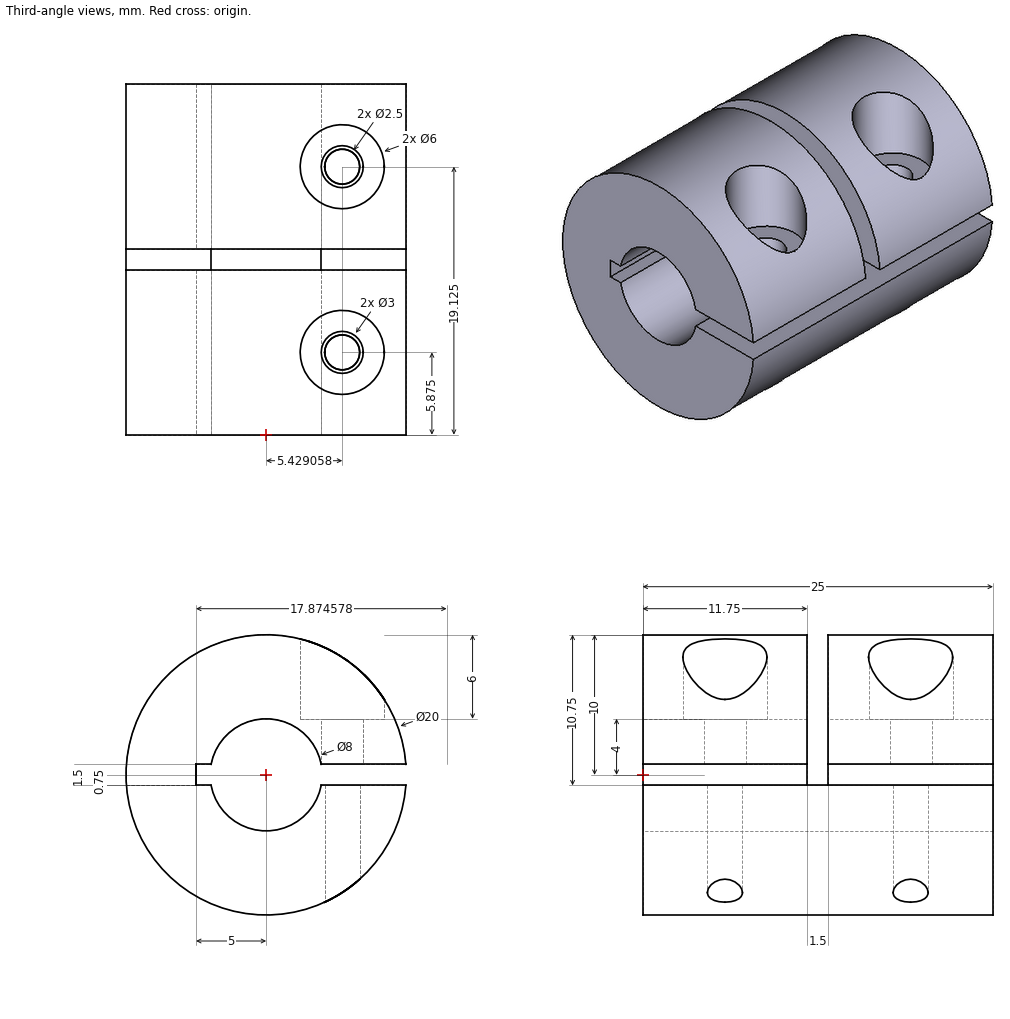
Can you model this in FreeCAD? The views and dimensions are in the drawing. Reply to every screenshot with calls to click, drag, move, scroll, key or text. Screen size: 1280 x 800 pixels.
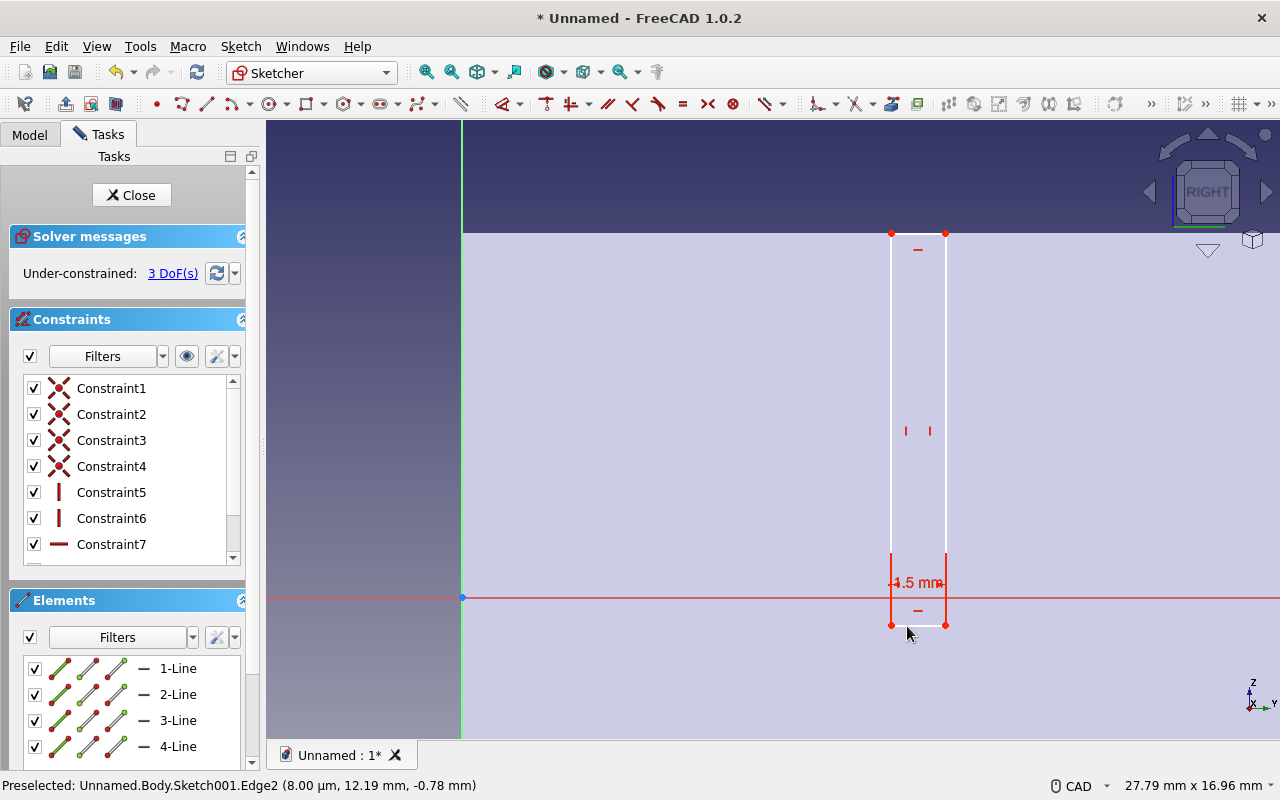
click(891, 234)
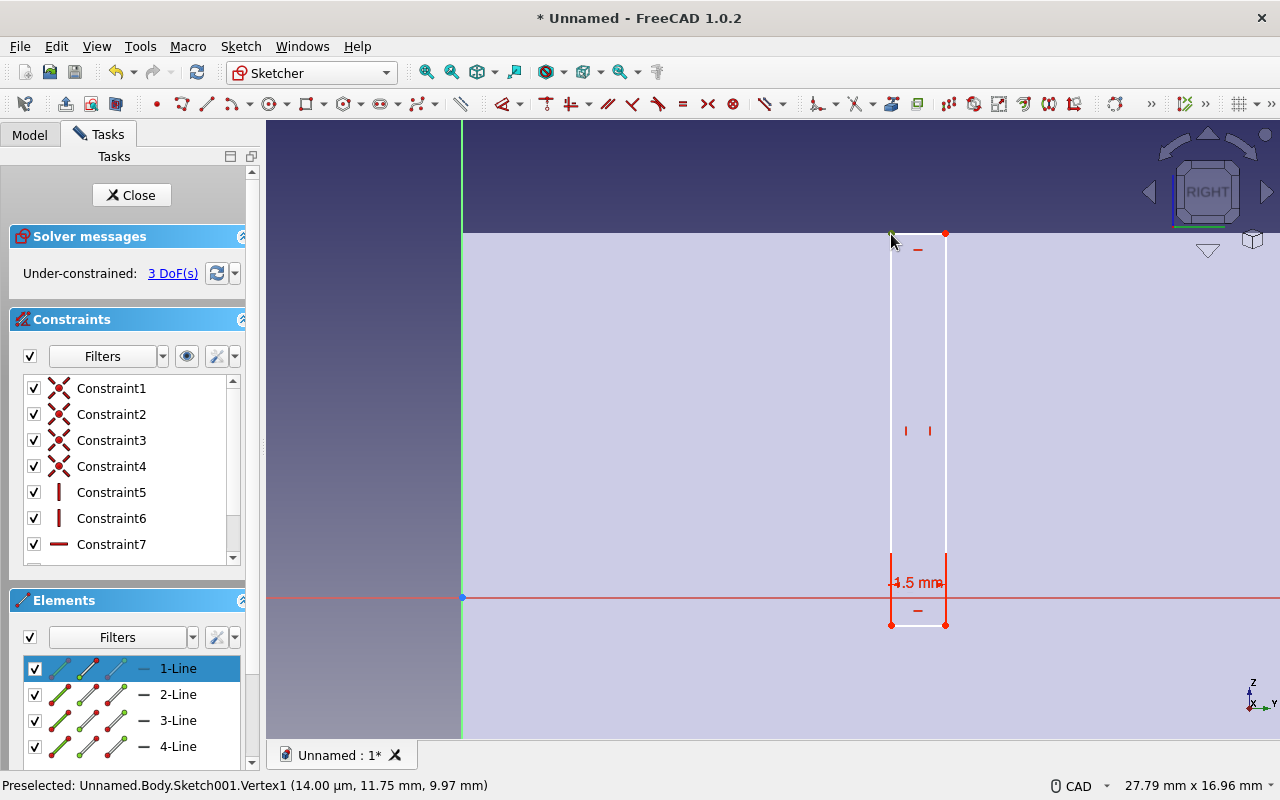
key(i)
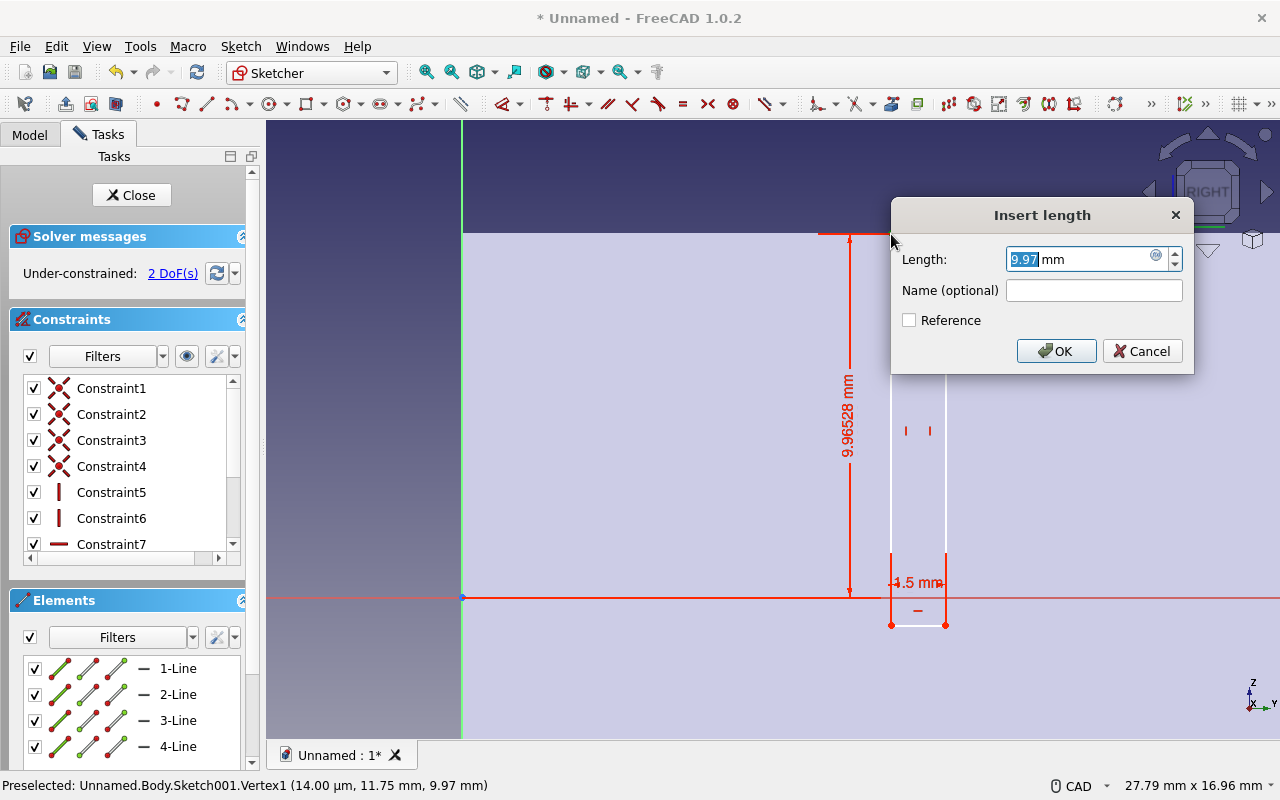
text(10)
key(Return)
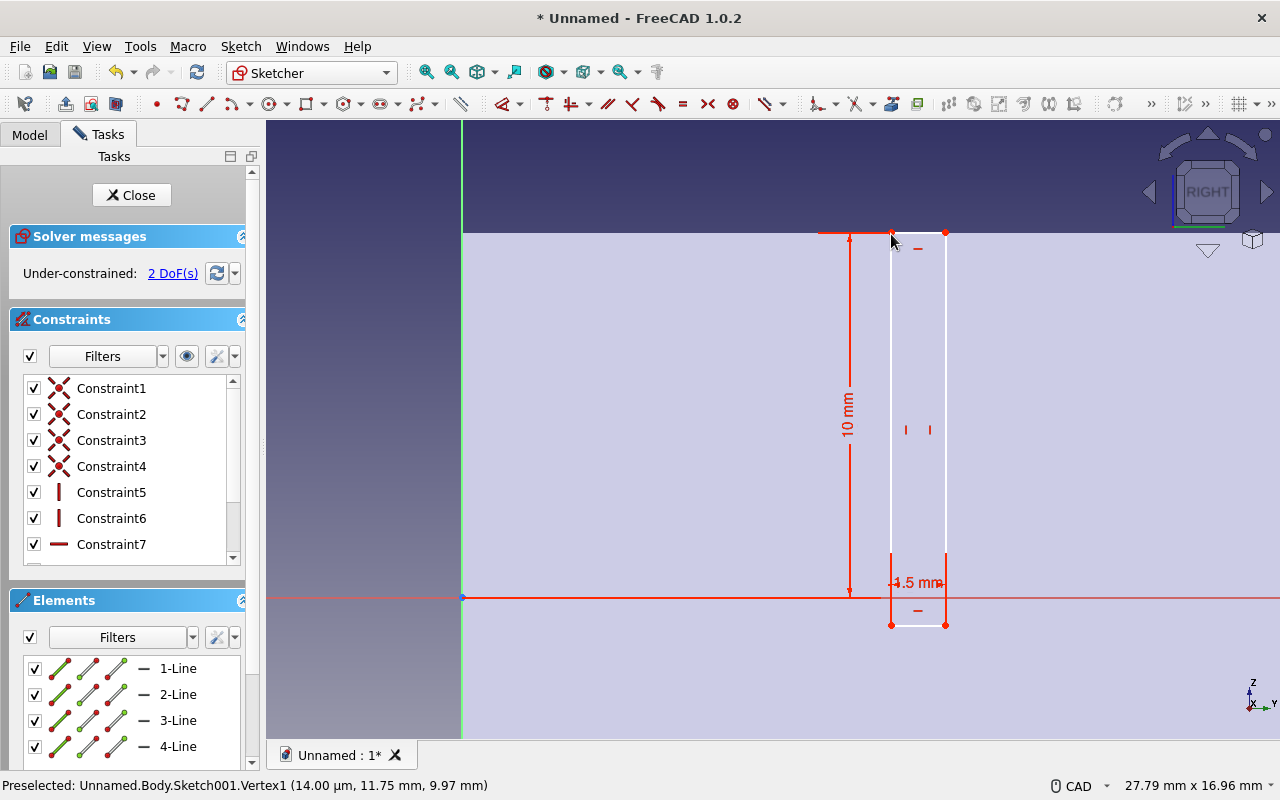
click(891, 351)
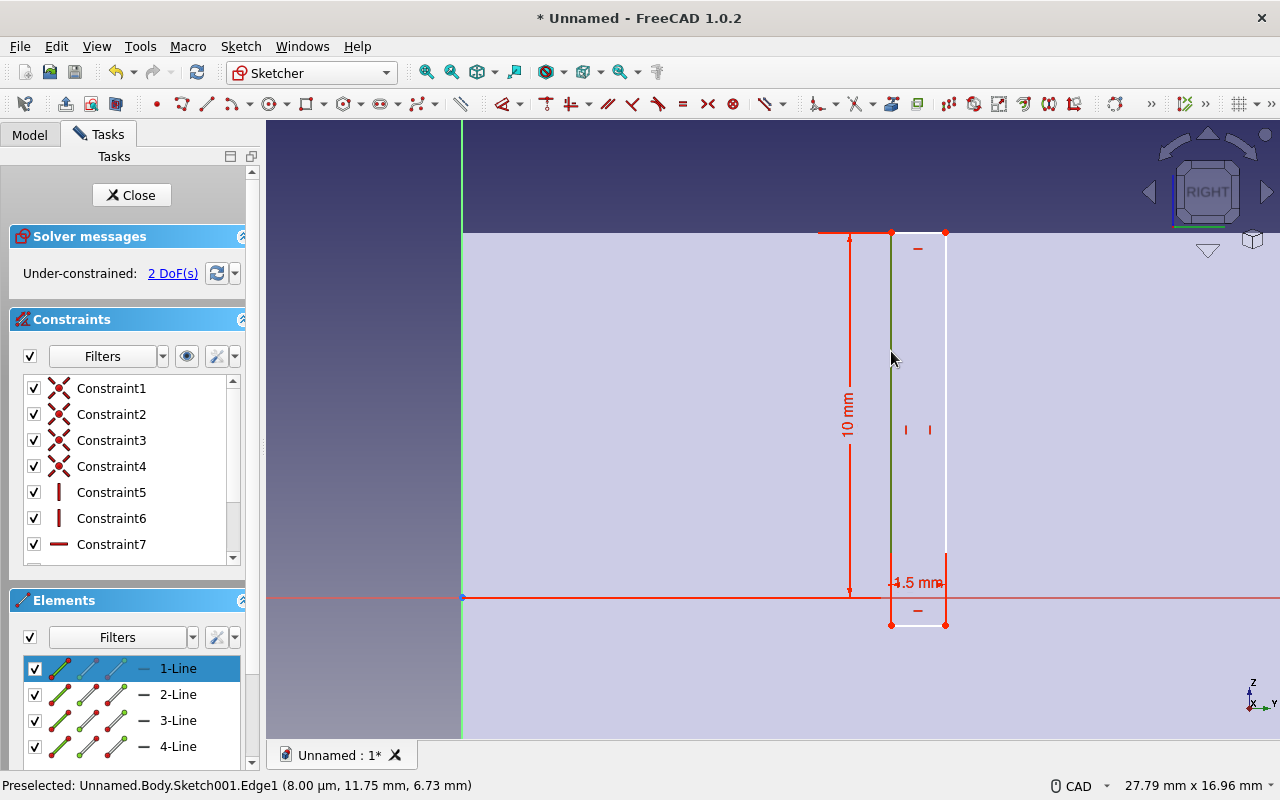
click(520, 104)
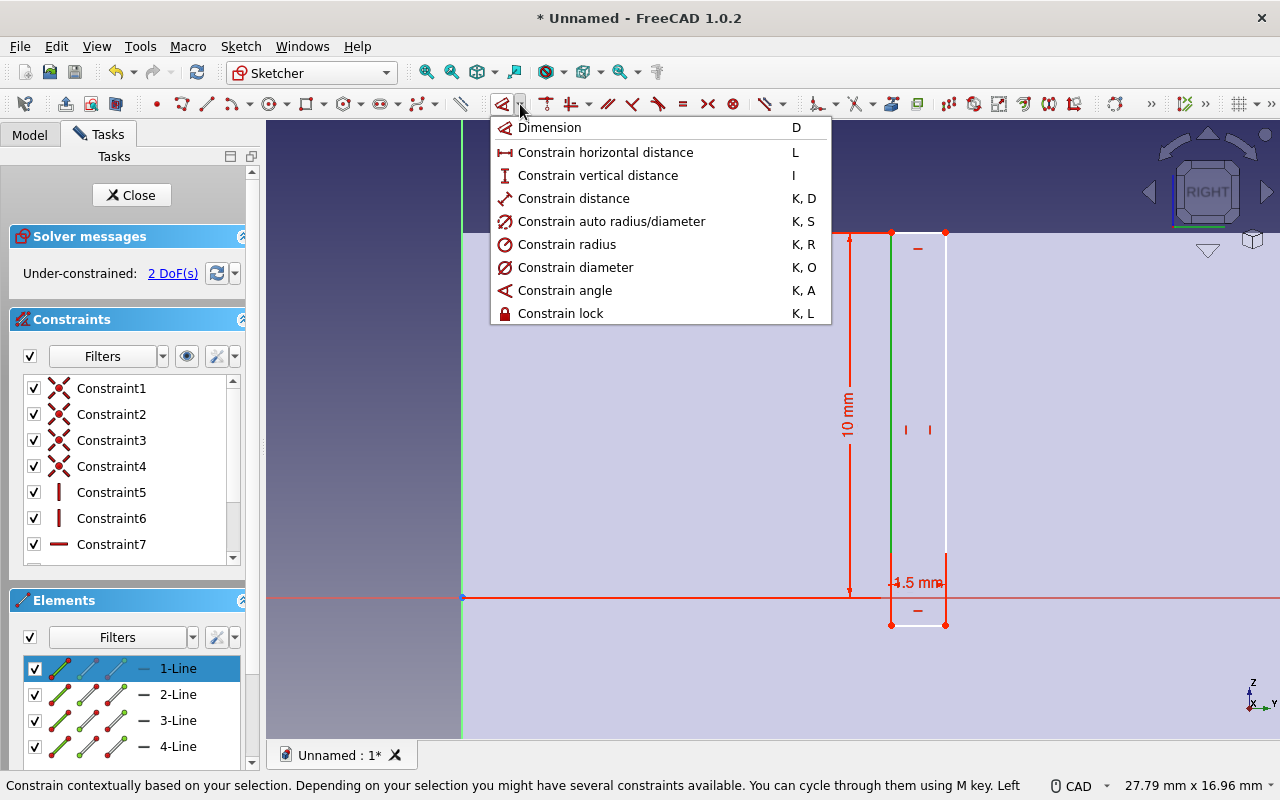
click(661, 176)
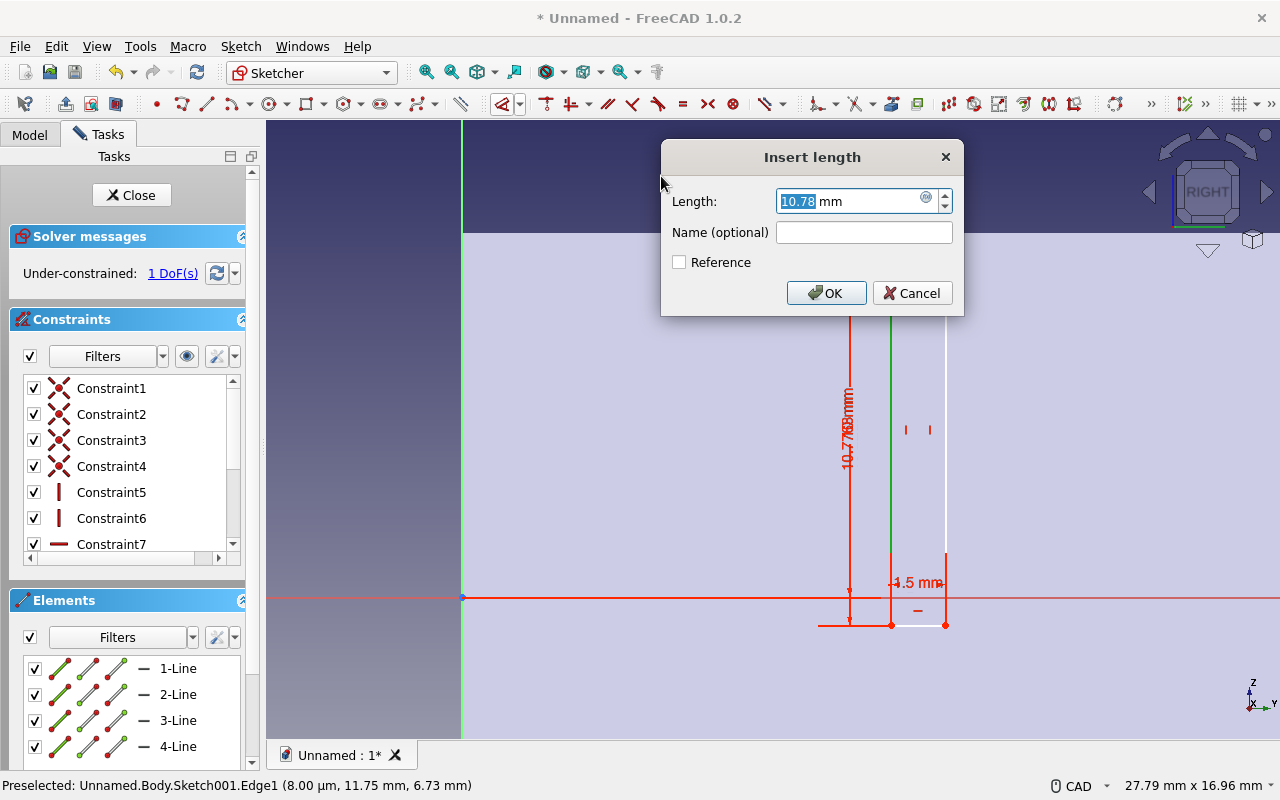
text(10.75)
key(Return)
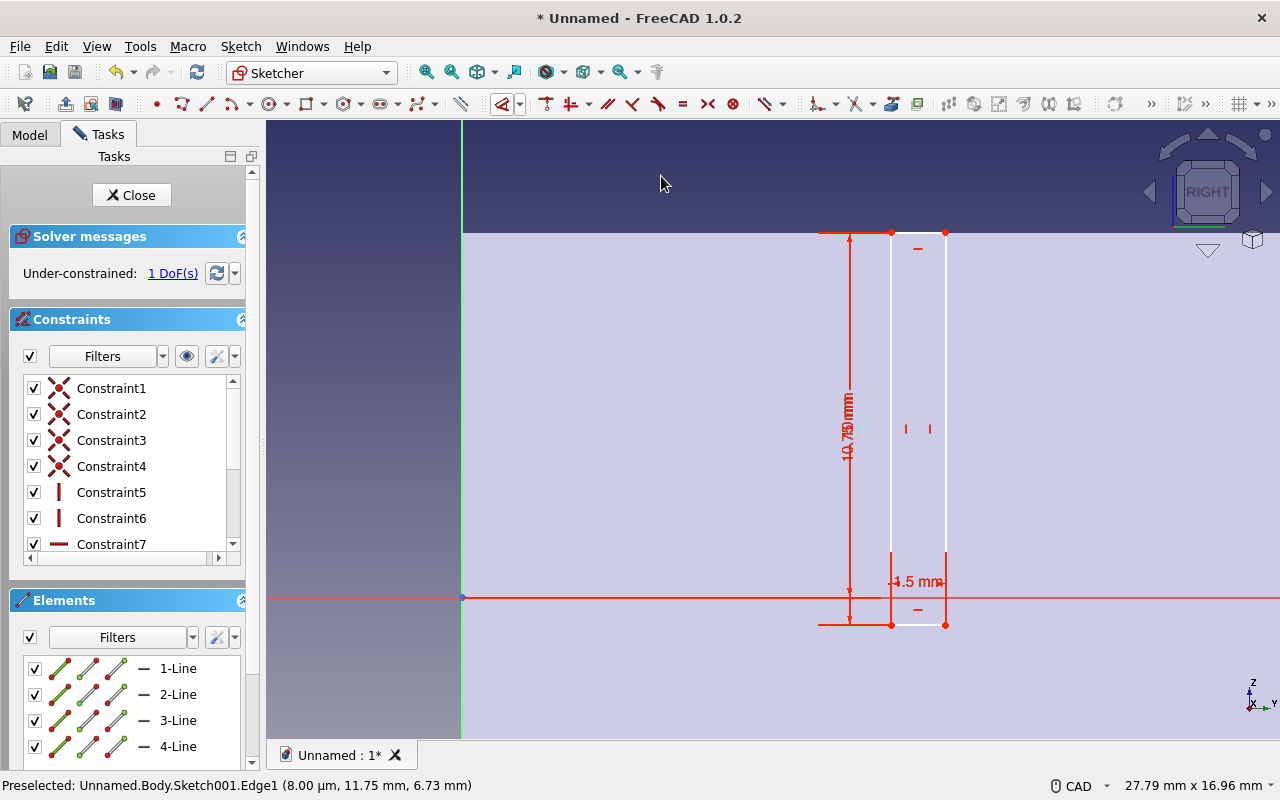
click(891, 233)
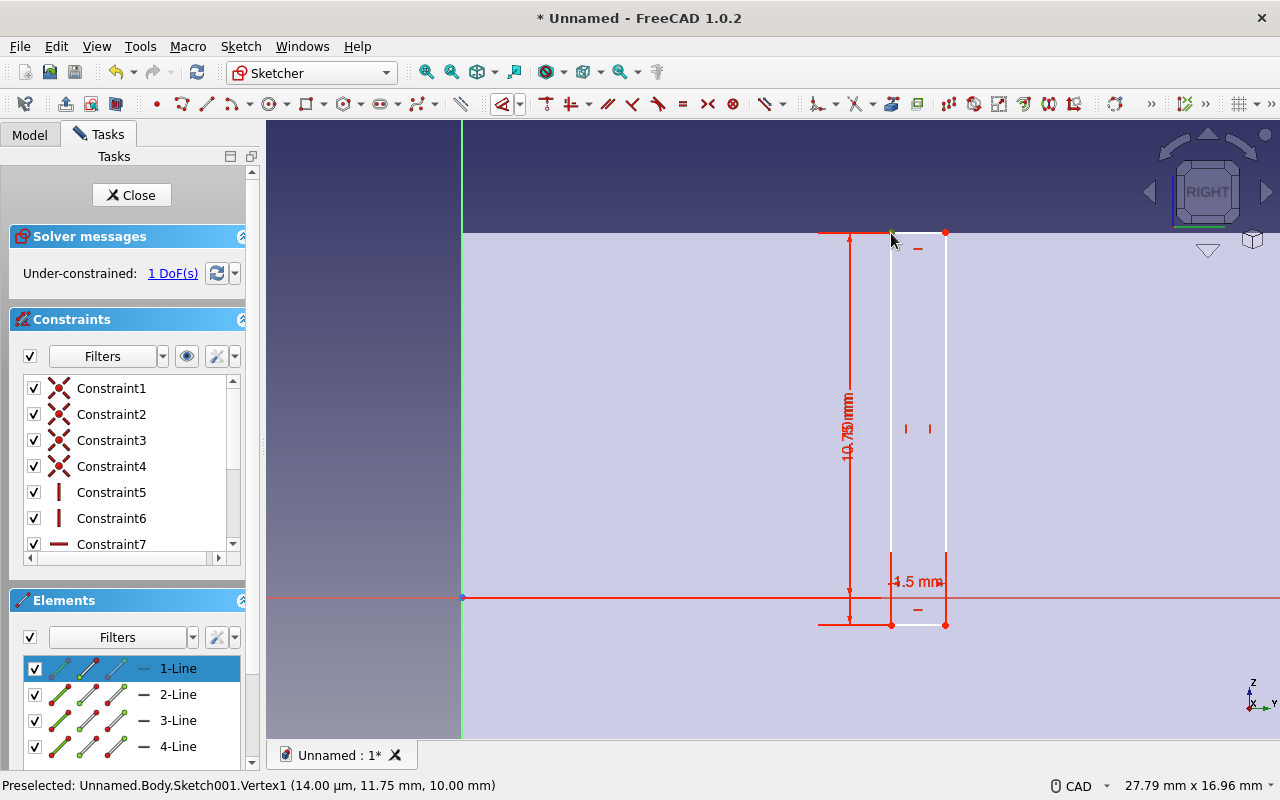
click(520, 104)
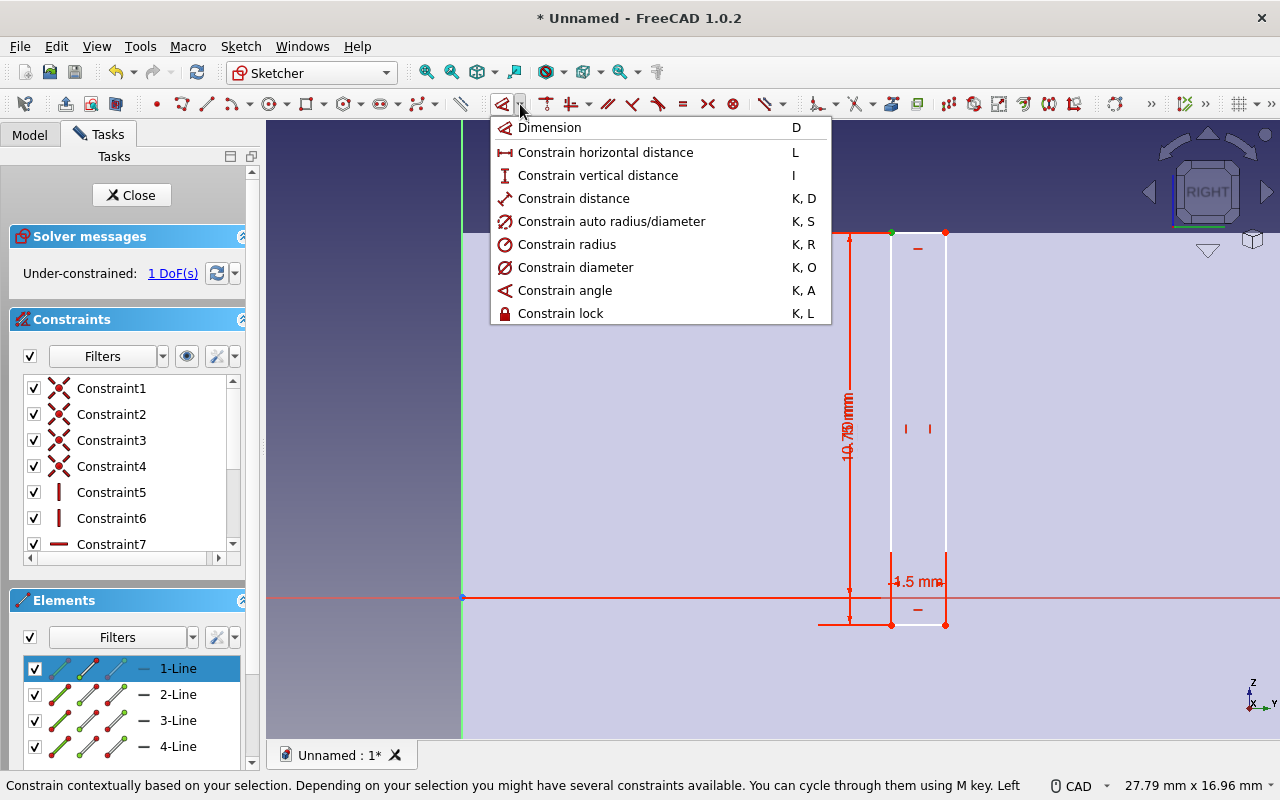
click(661, 152)